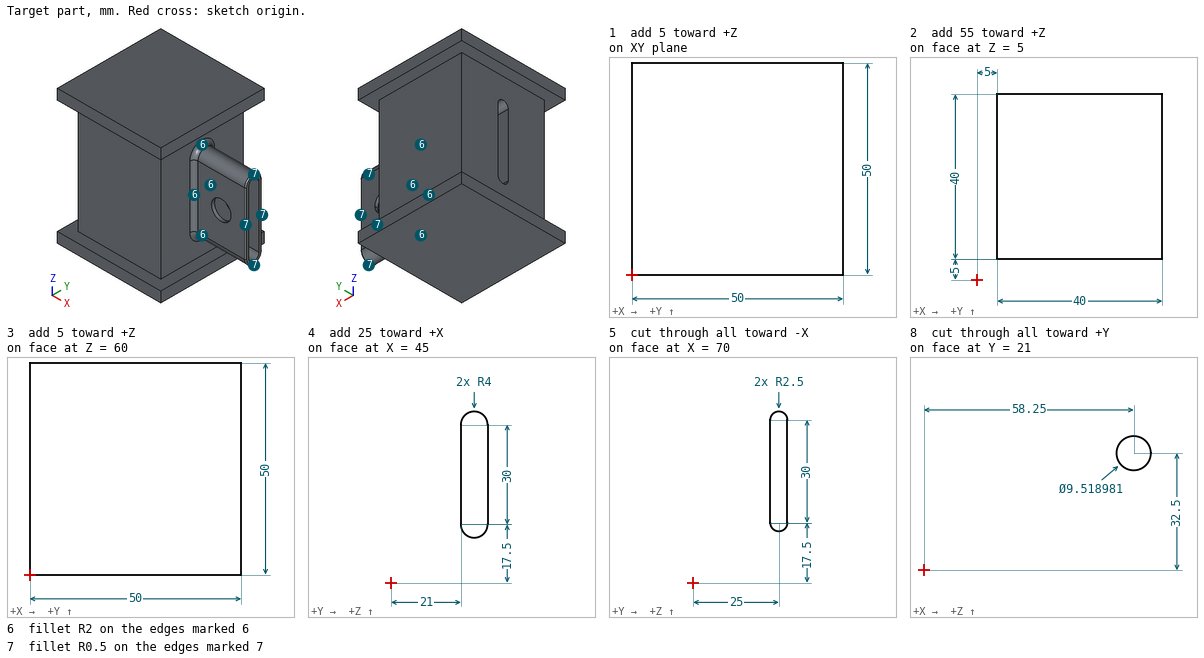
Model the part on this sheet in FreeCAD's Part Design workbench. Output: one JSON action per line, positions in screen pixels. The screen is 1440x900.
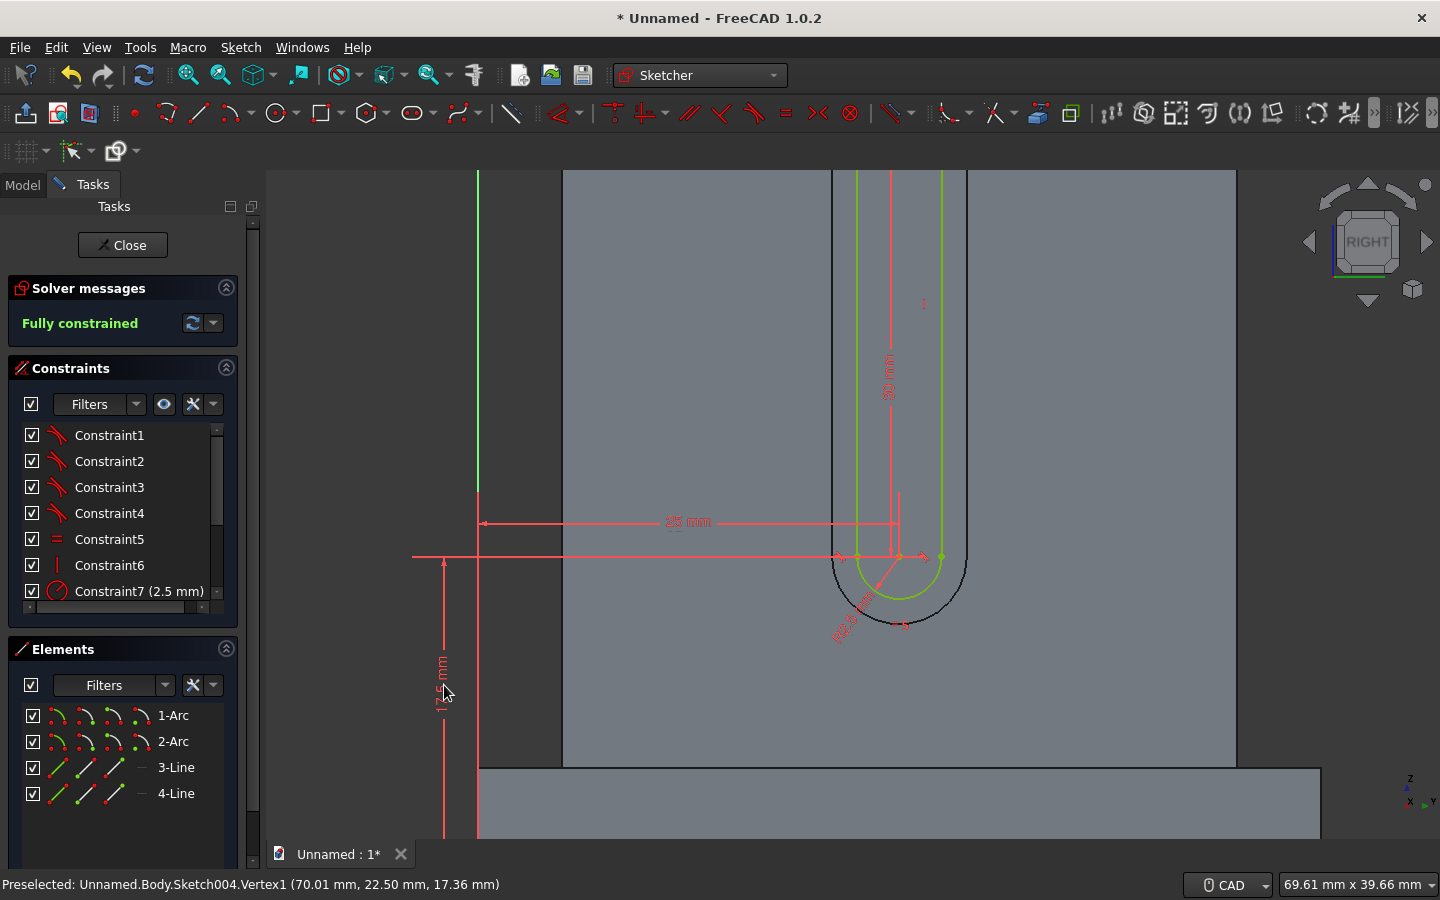
{"action": "left_click", "coordinate": [123, 245]}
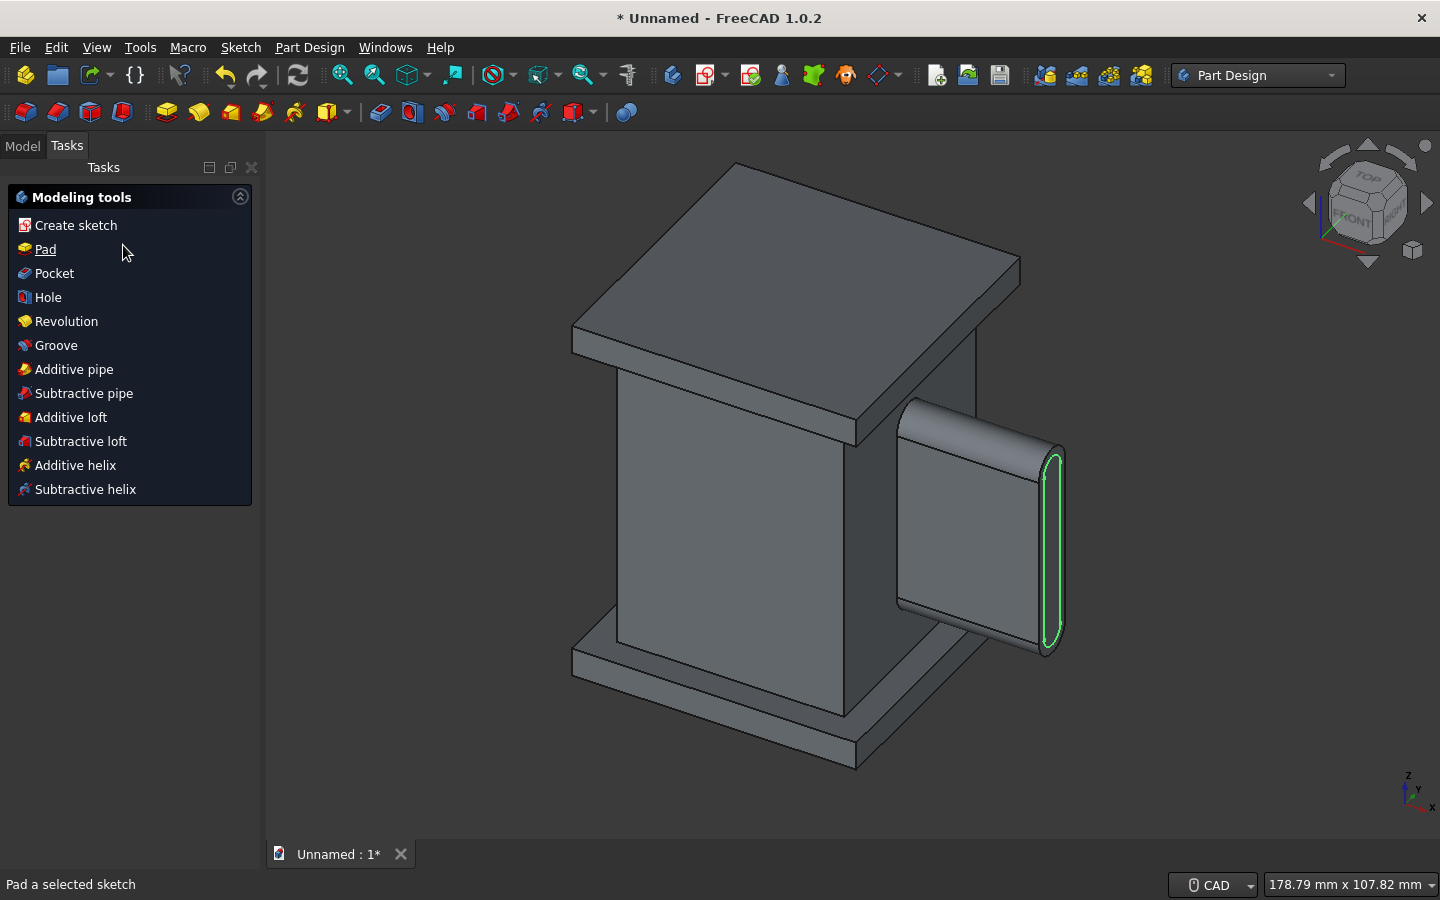
{"action": "left_click", "coordinate": [382, 112]}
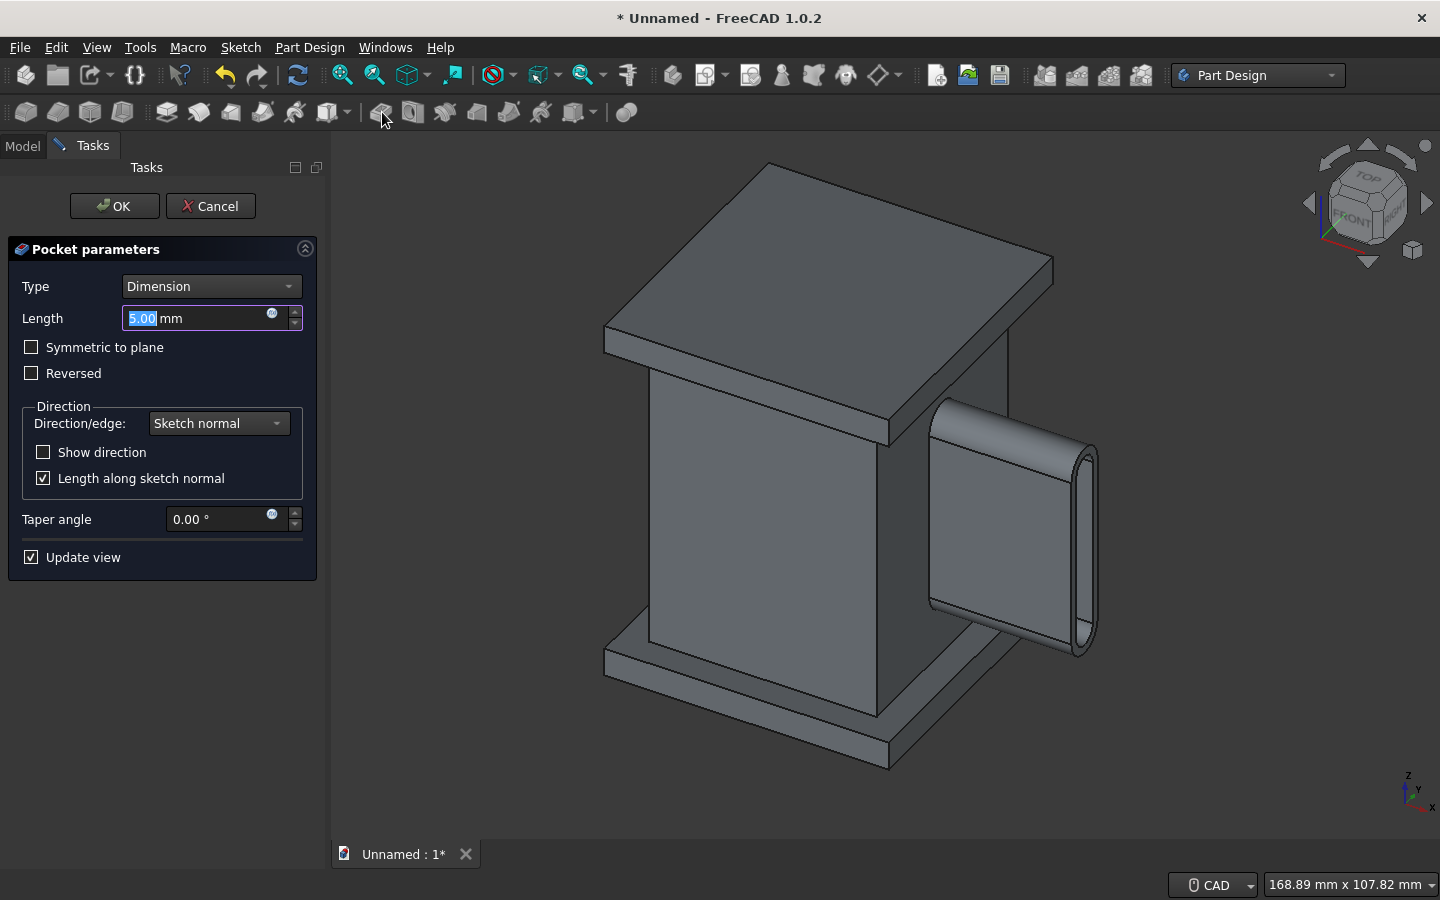
{"action": "left_click", "coordinate": [212, 286]}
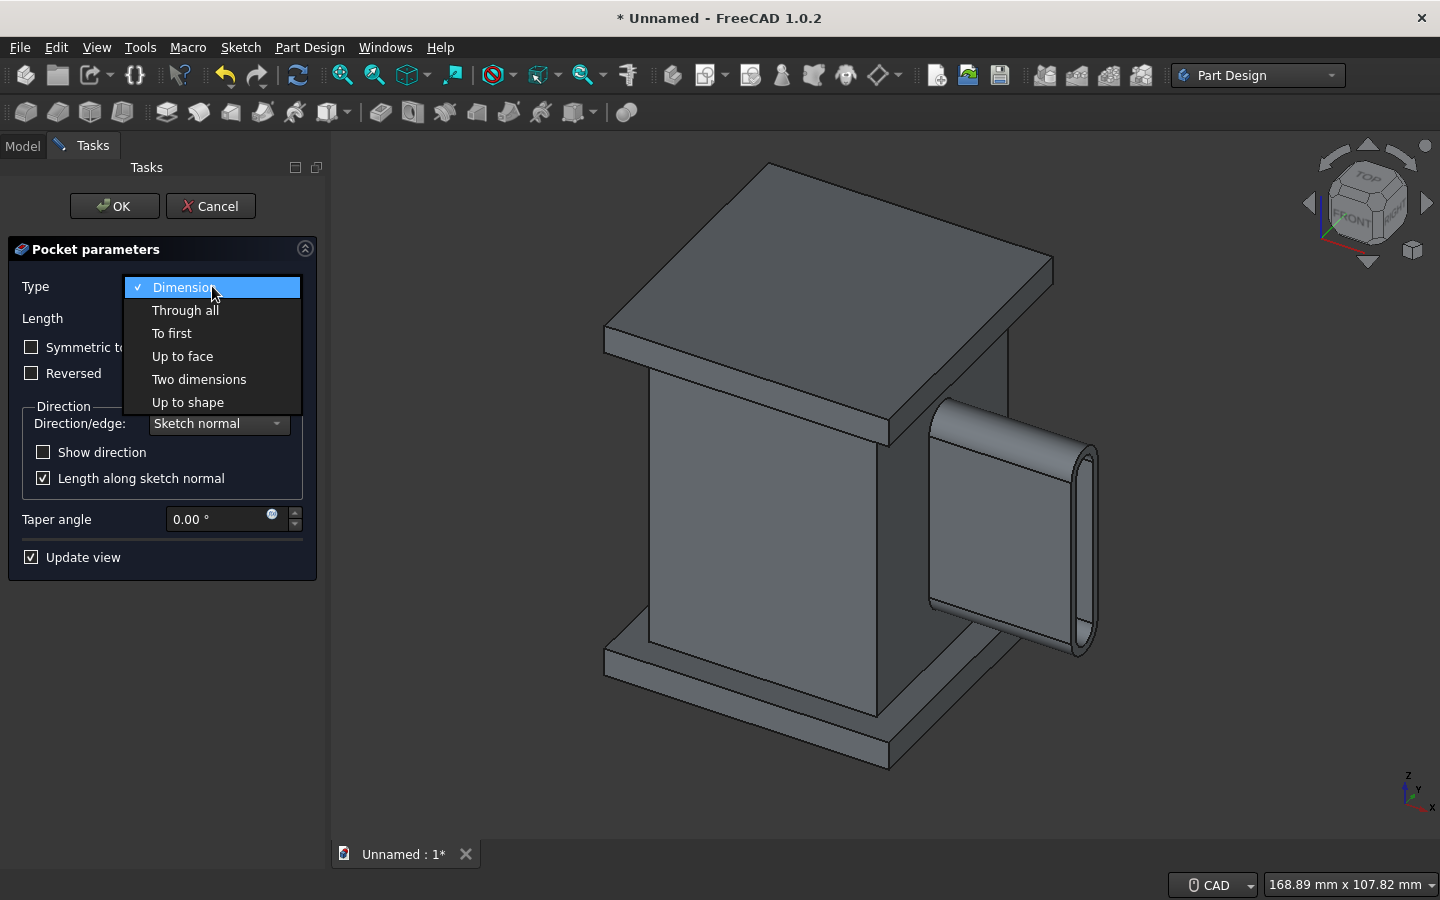
{"action": "left_click", "coordinate": [212, 310]}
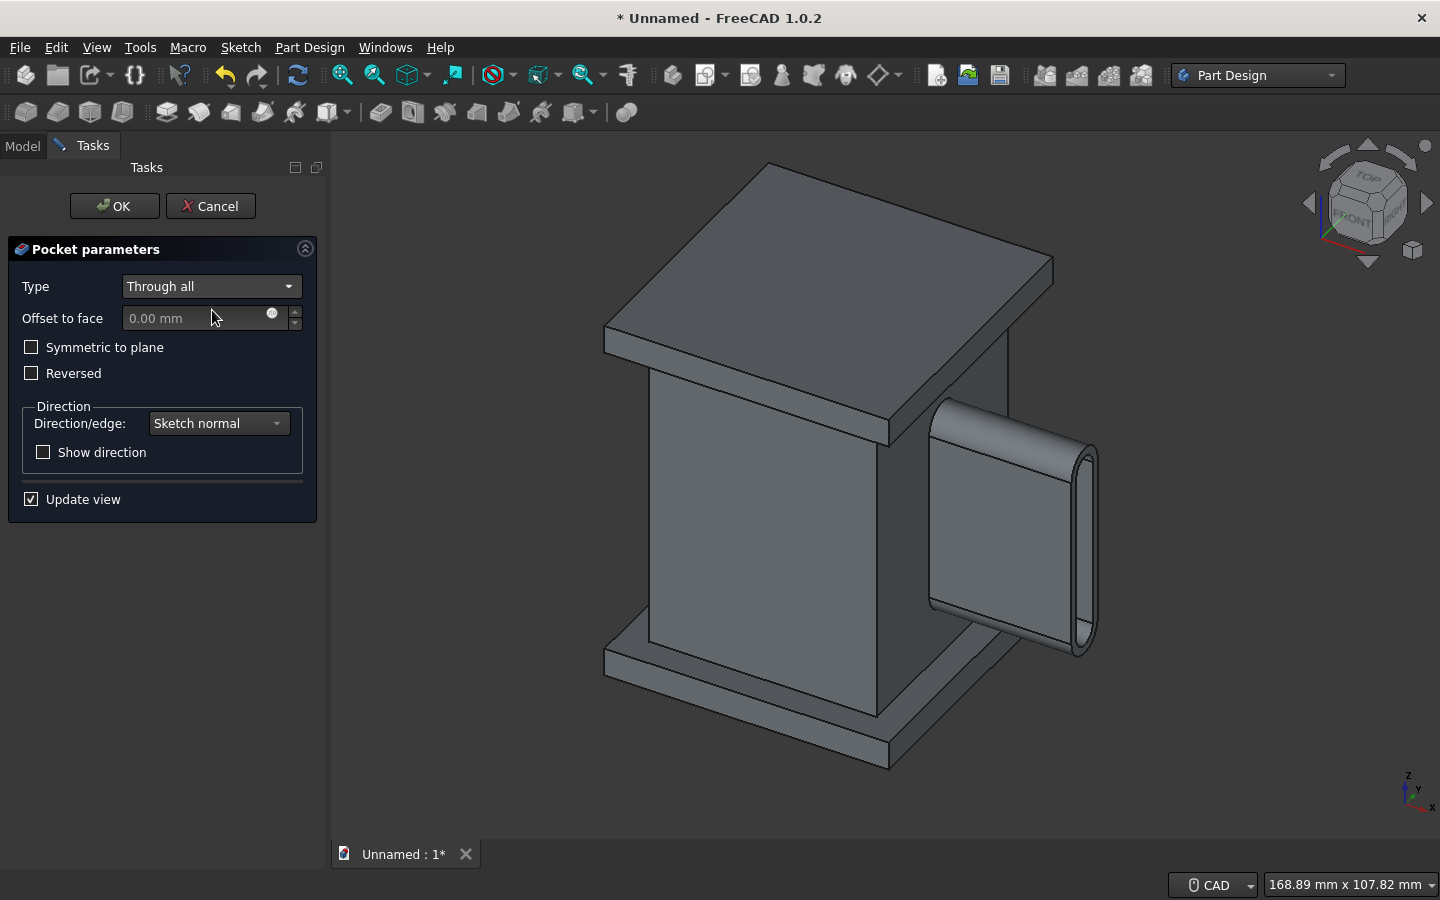
{"action": "left_click", "coordinate": [115, 206]}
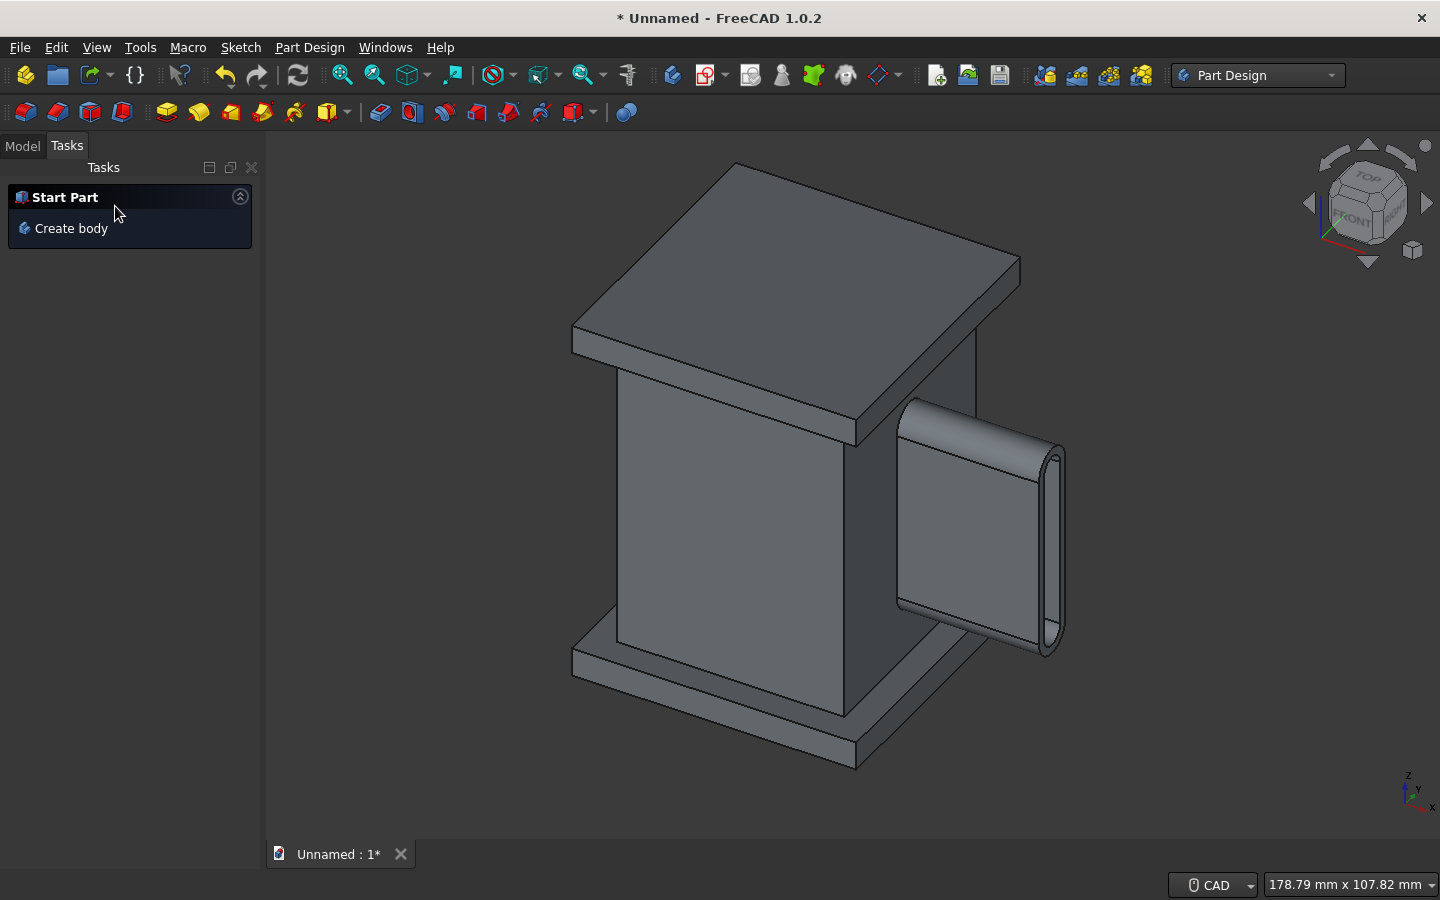
{"action": "left_click", "coordinate": [899, 607]}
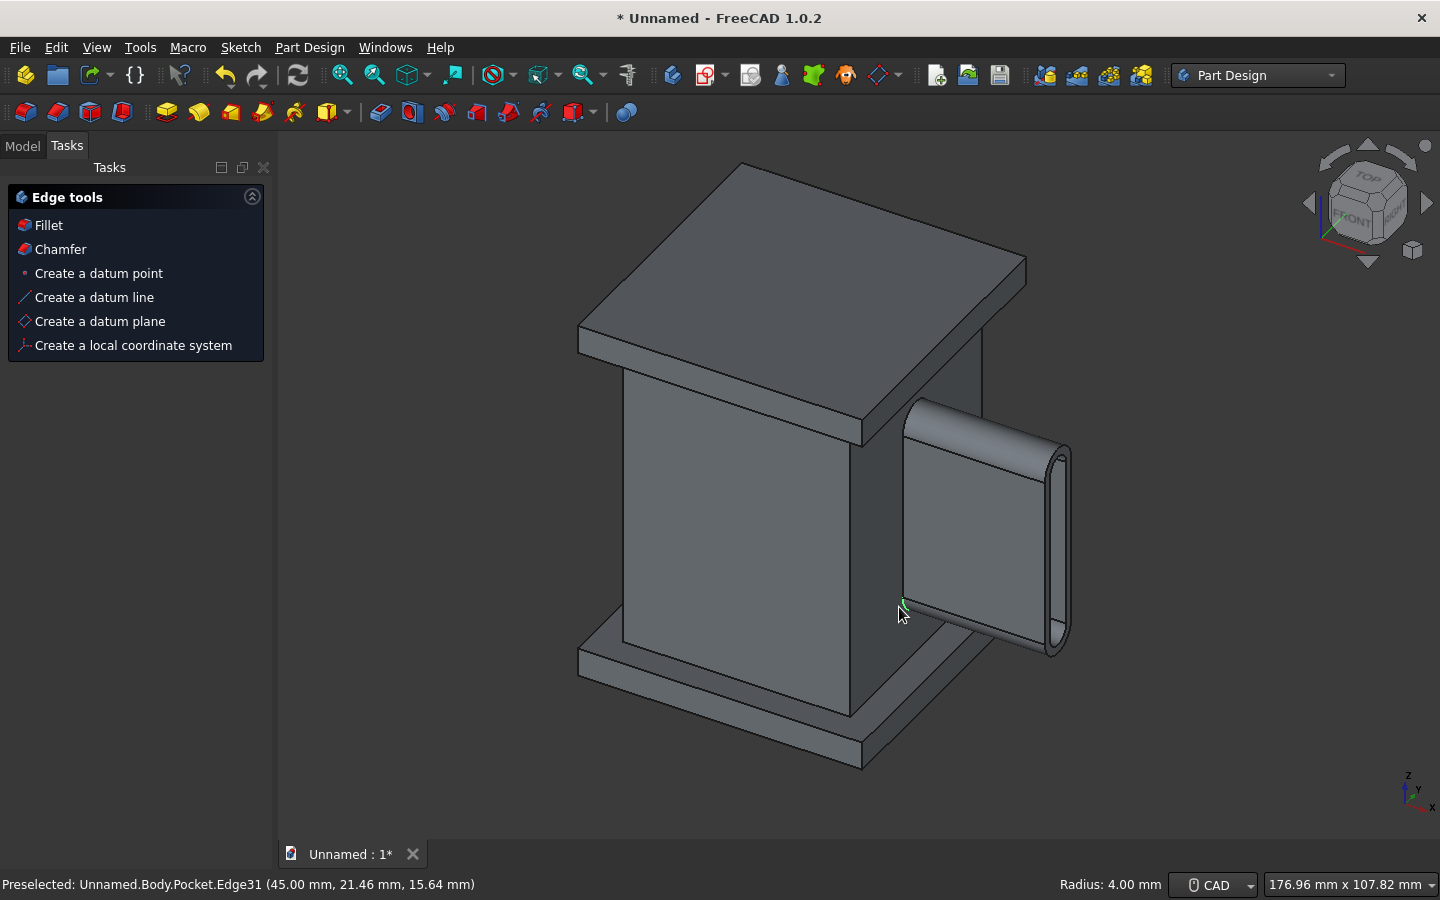
{"action": "left_click", "coordinate": [920, 398], "text": "ctrl"}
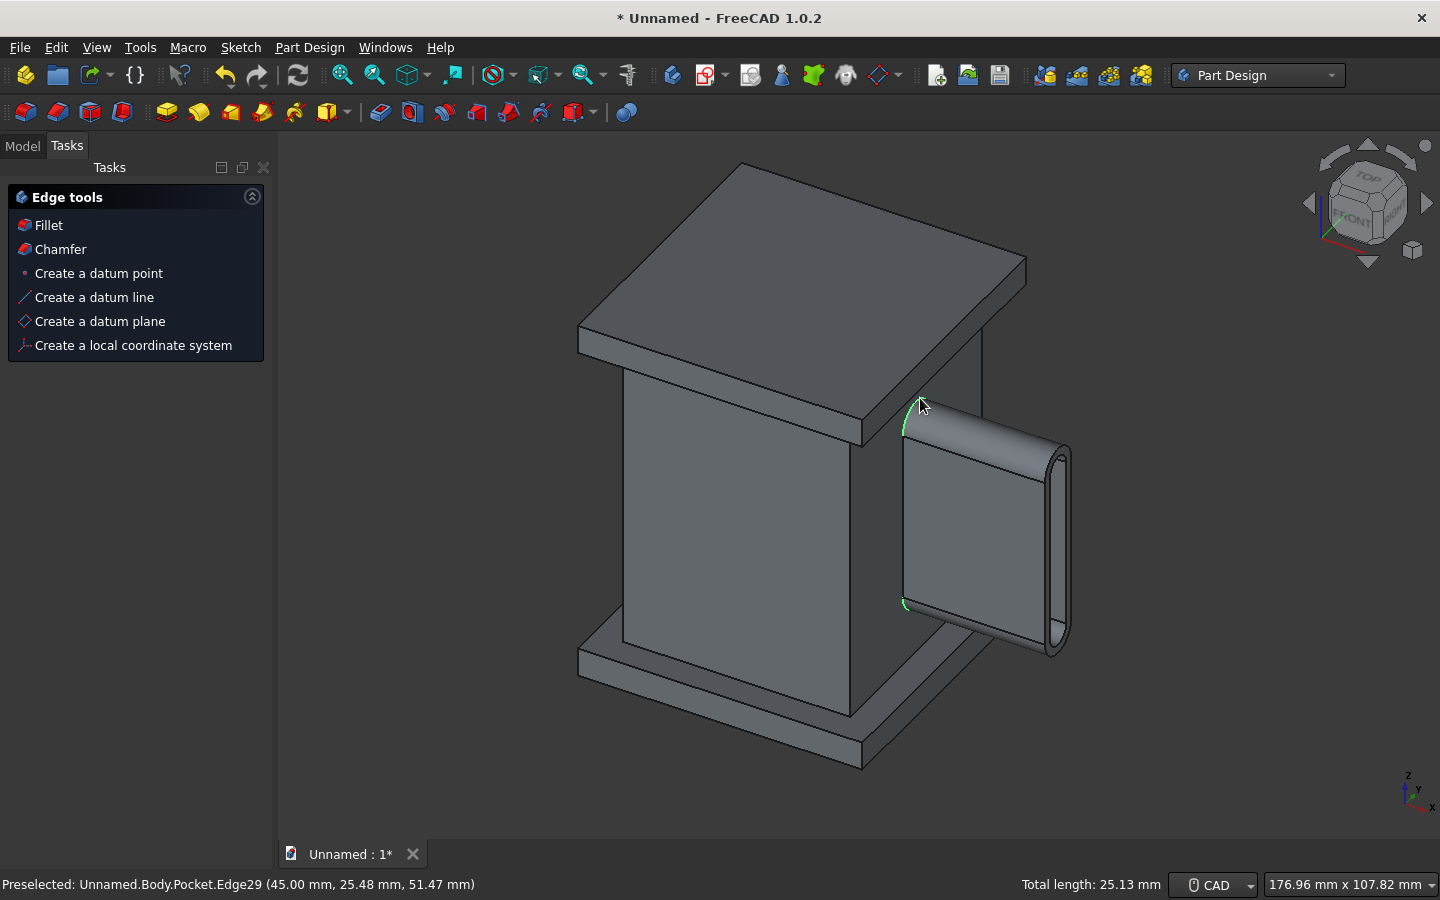
{"action": "key", "text": "0"}